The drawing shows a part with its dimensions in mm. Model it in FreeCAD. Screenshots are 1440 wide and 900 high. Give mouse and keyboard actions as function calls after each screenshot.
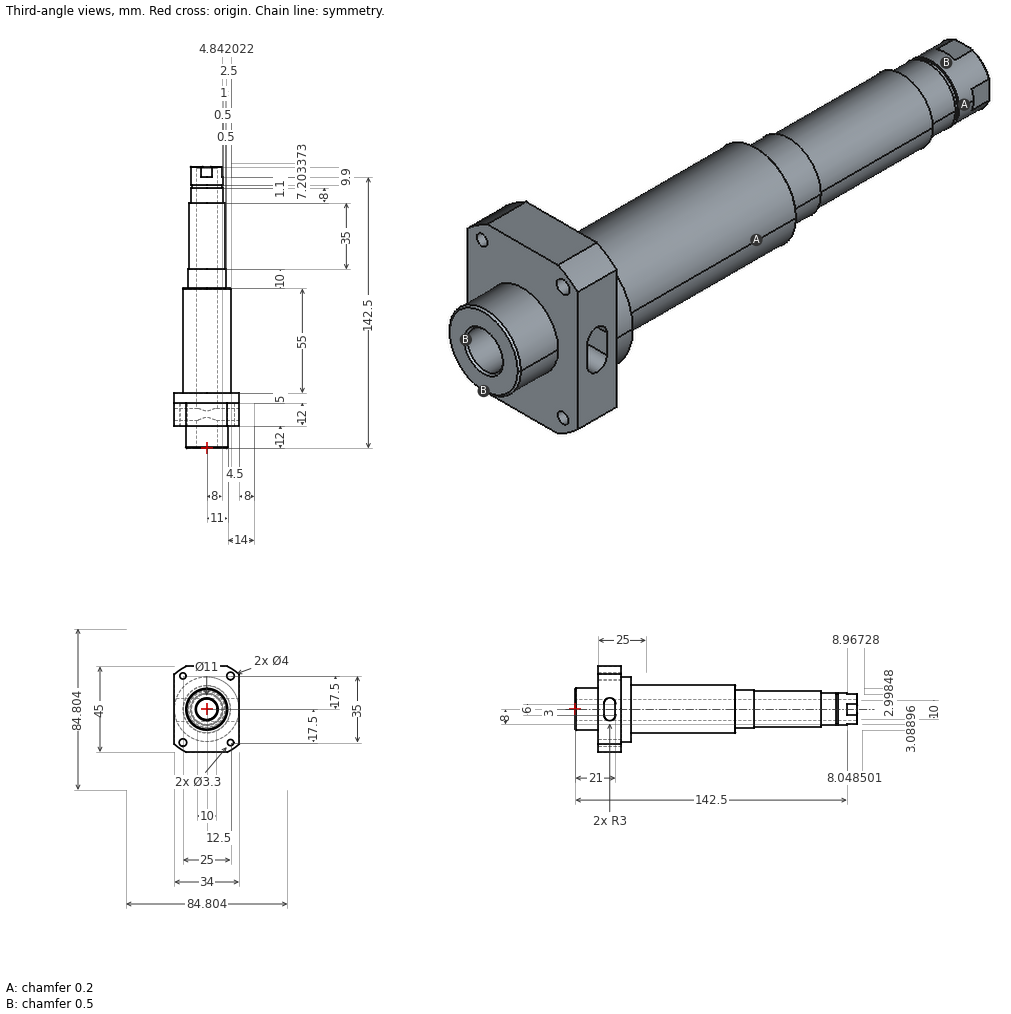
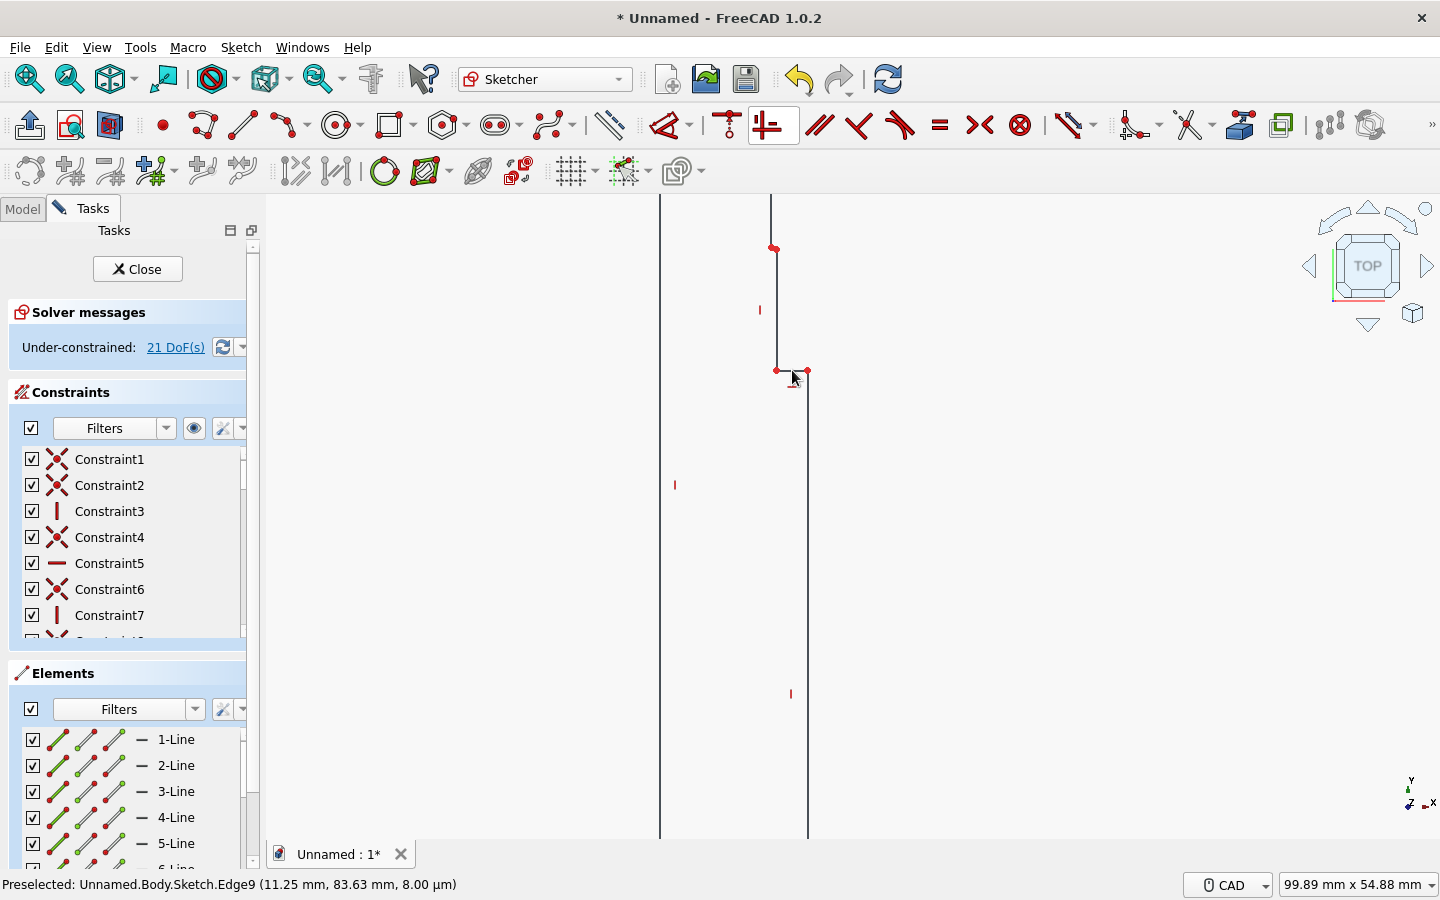
scroll(774, 248, up, 7)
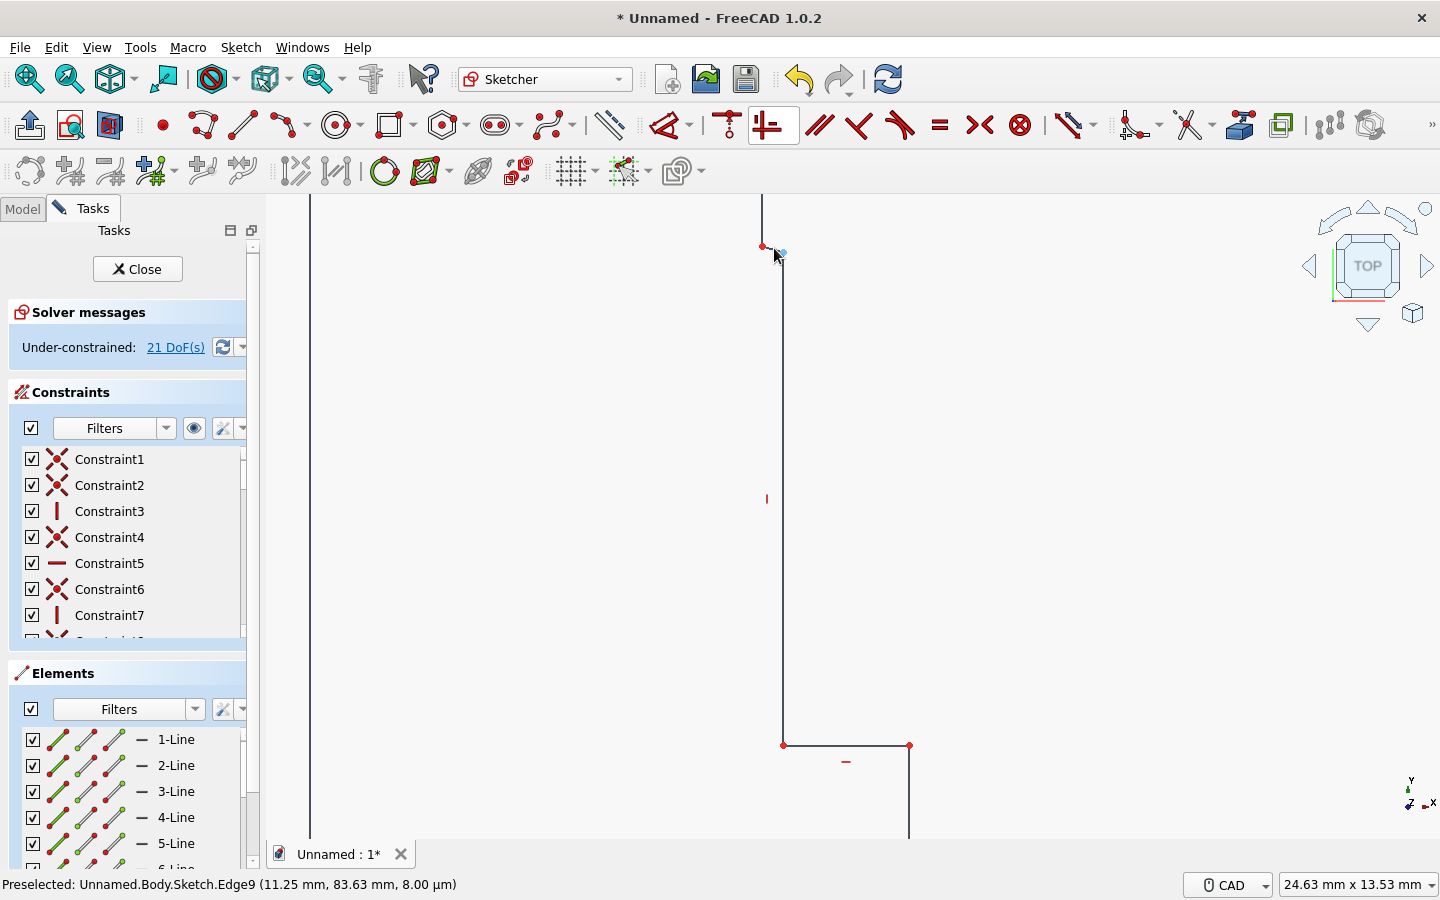
click(773, 249)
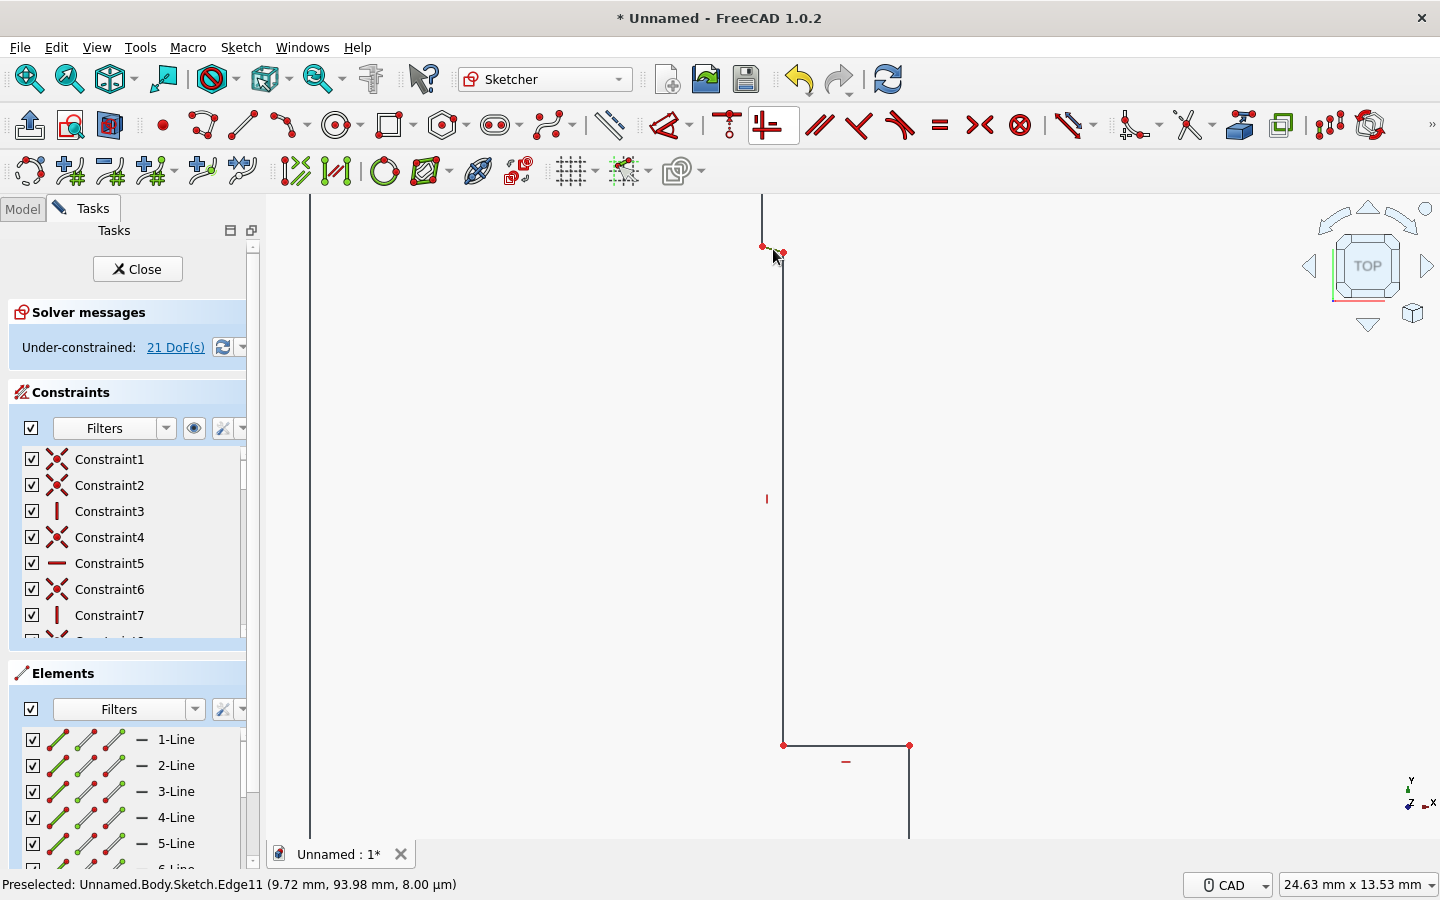
key(h)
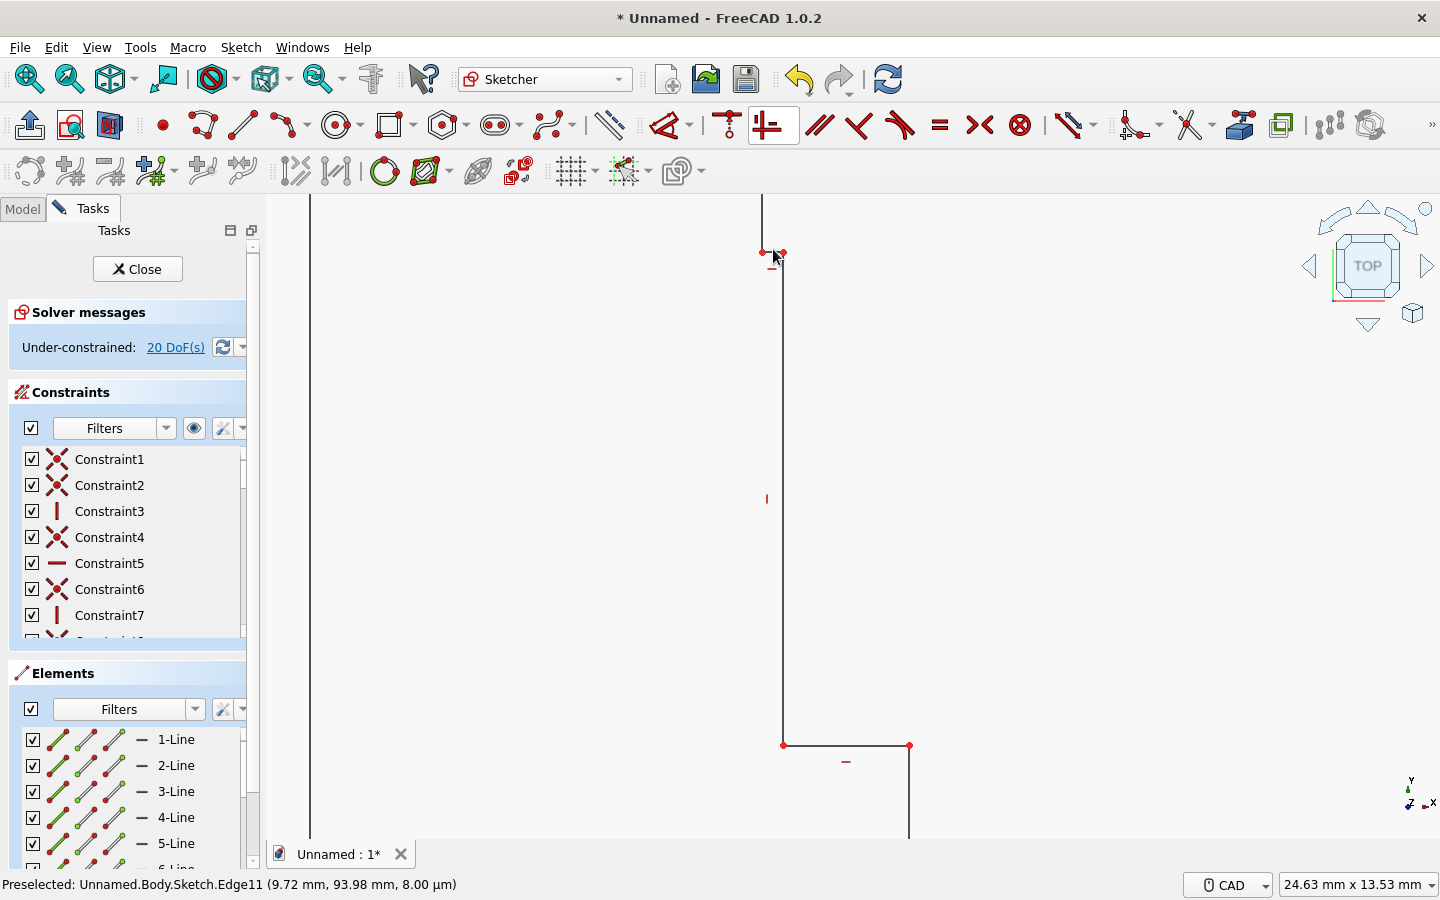
scroll(777, 472, down, 14)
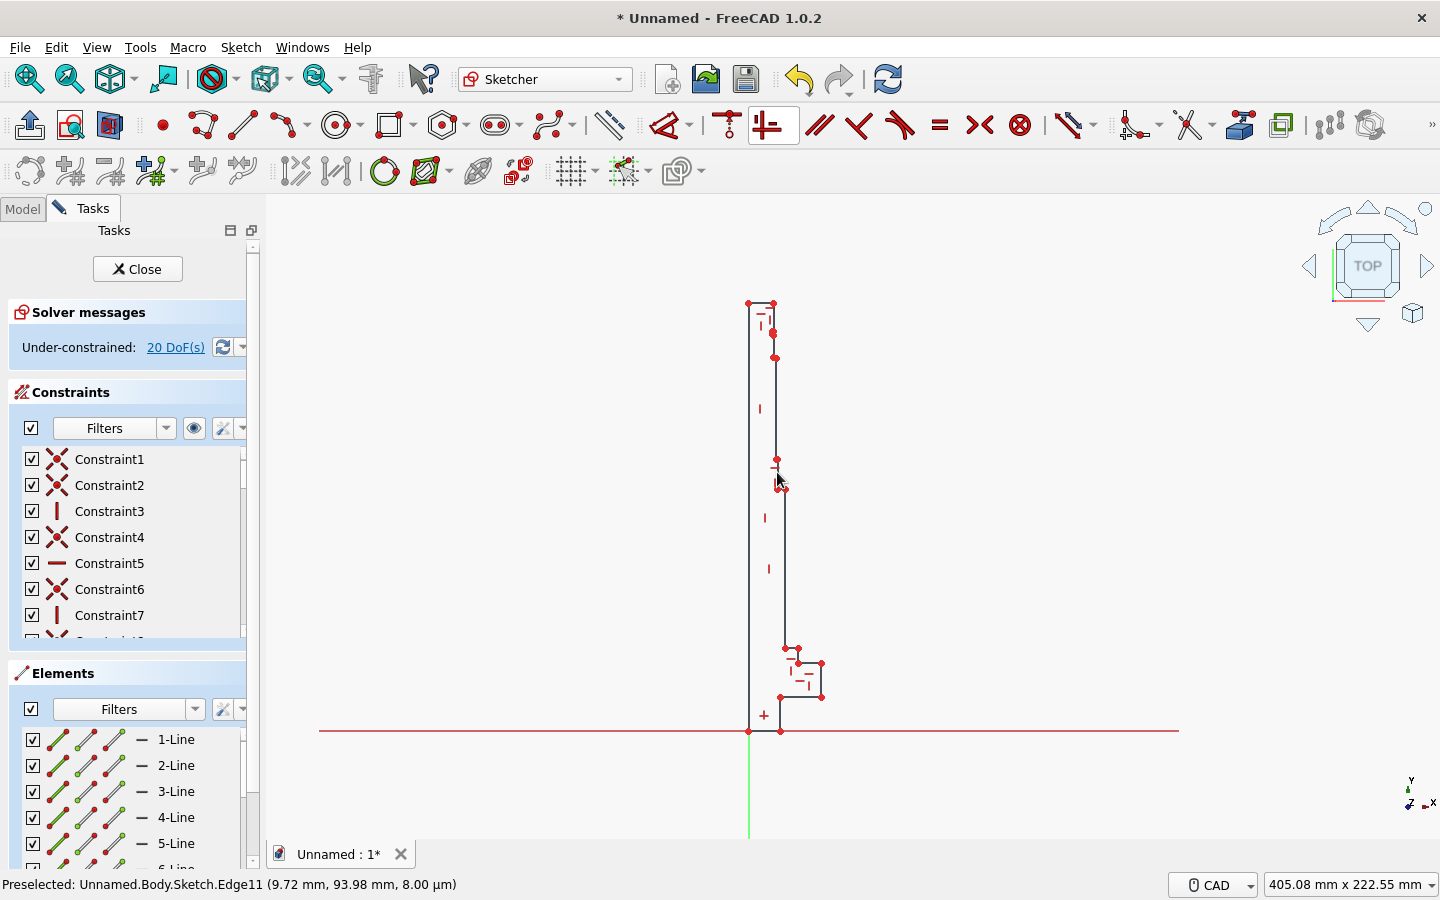
scroll(776, 358, up, 14)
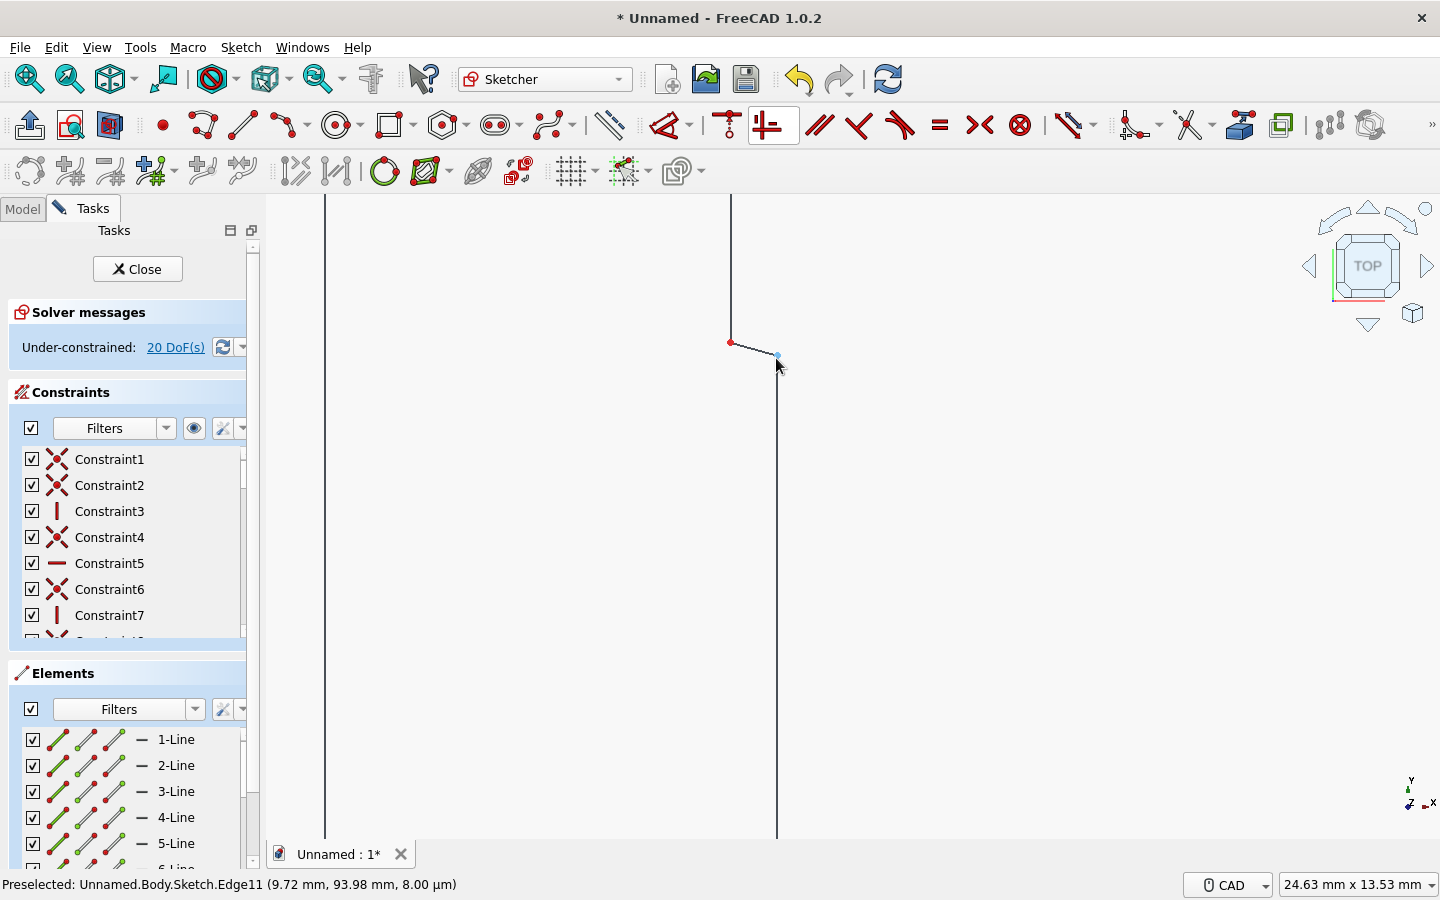
click(763, 352)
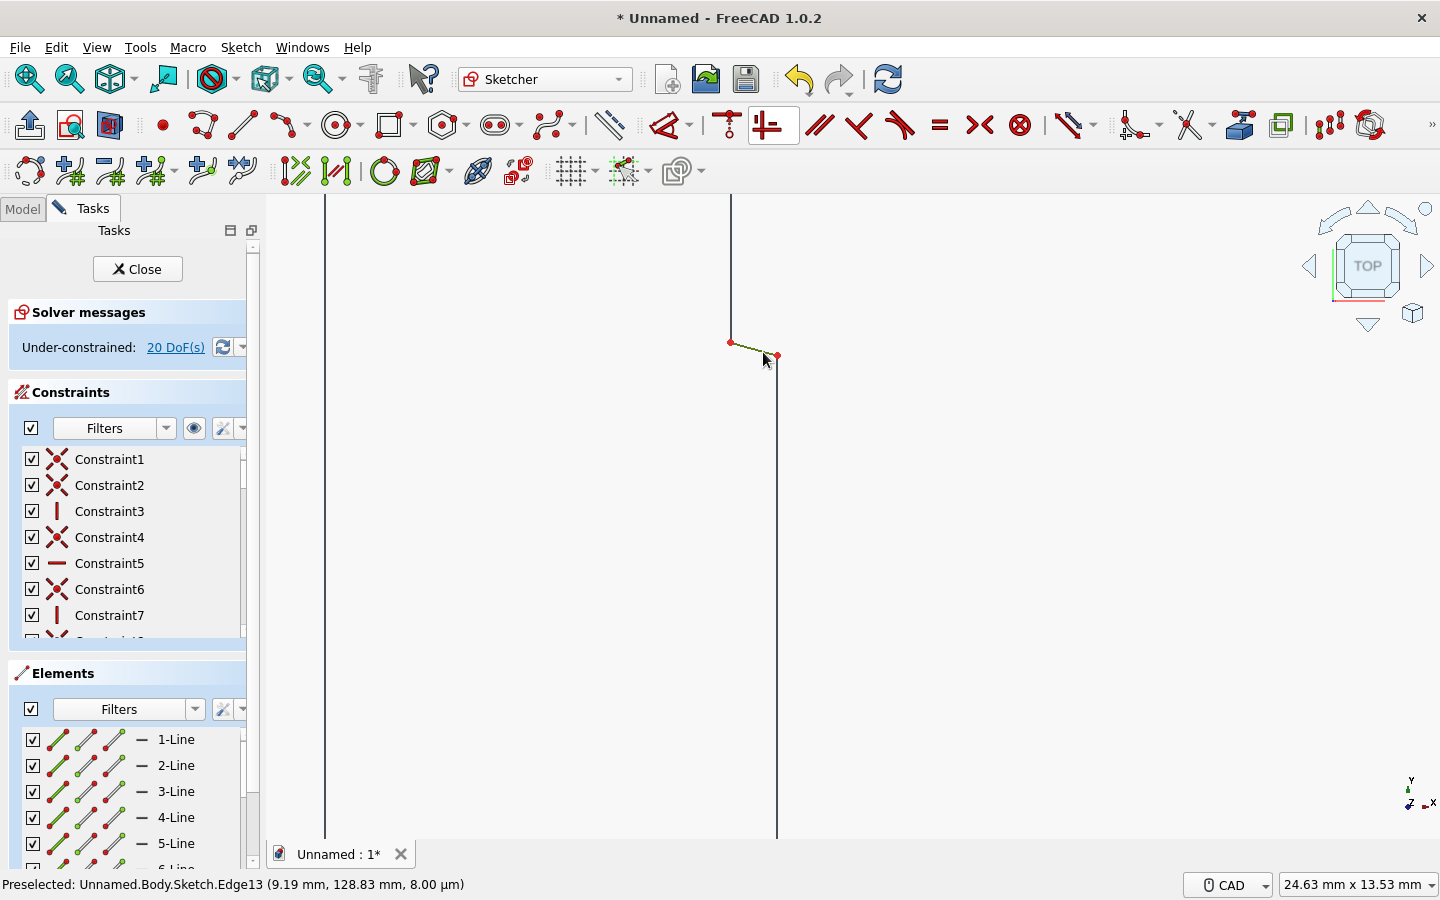
click(794, 126)